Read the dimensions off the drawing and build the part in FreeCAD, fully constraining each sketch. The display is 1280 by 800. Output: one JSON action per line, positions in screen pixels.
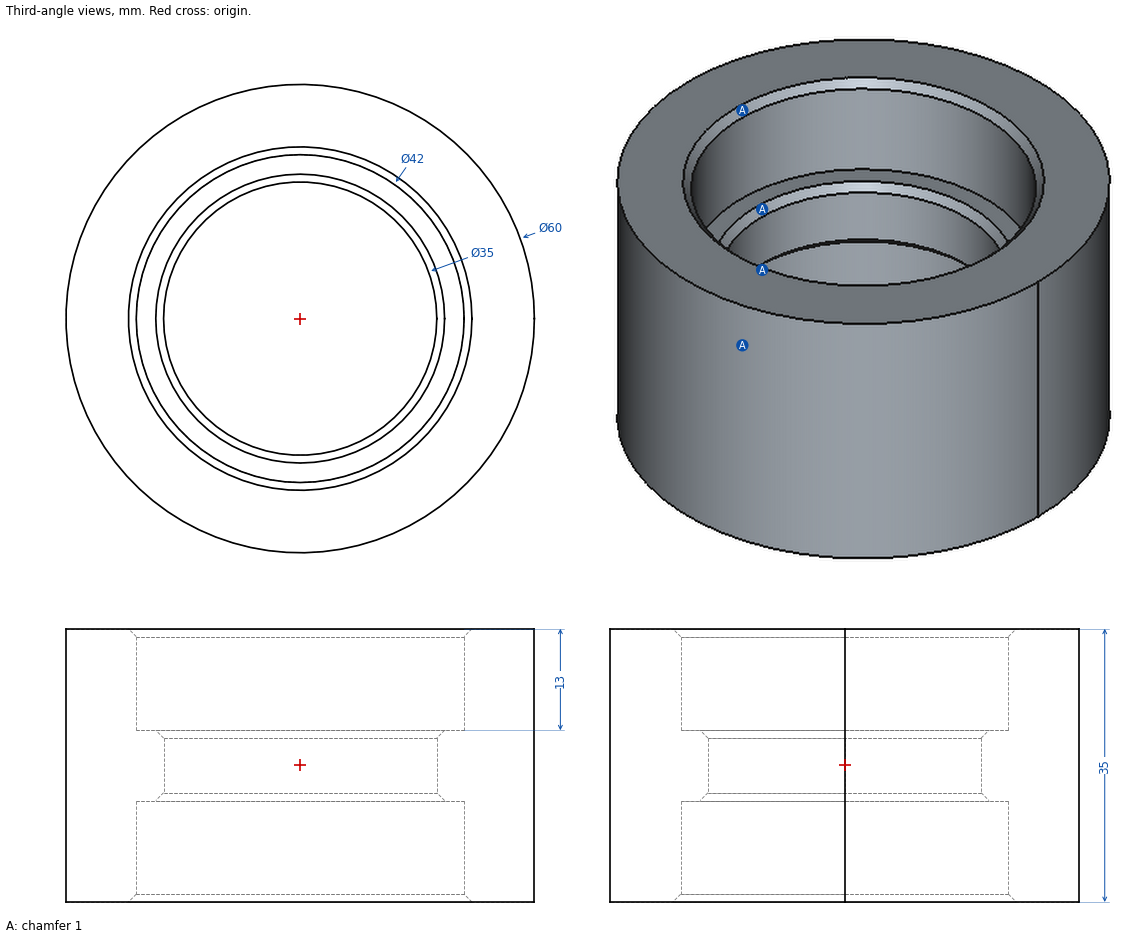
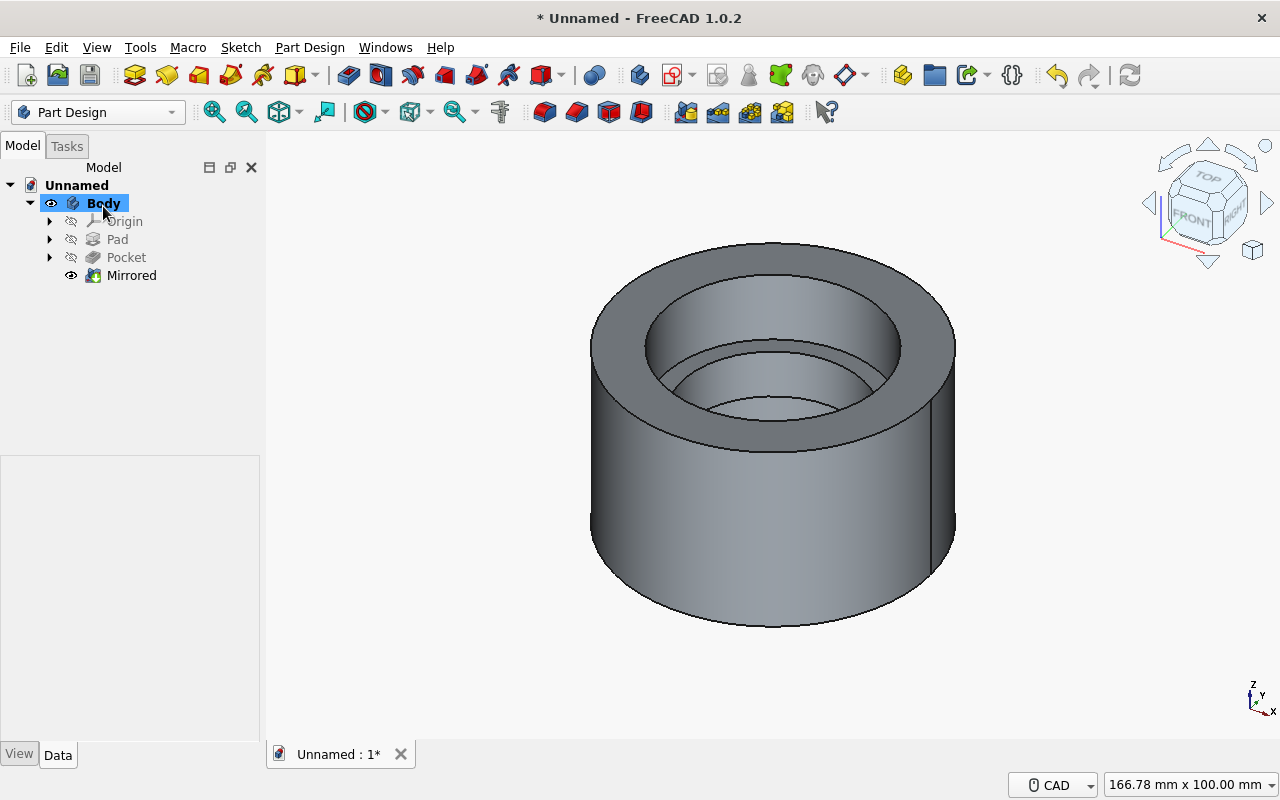
{"action": "left_click", "coordinate": [681, 381]}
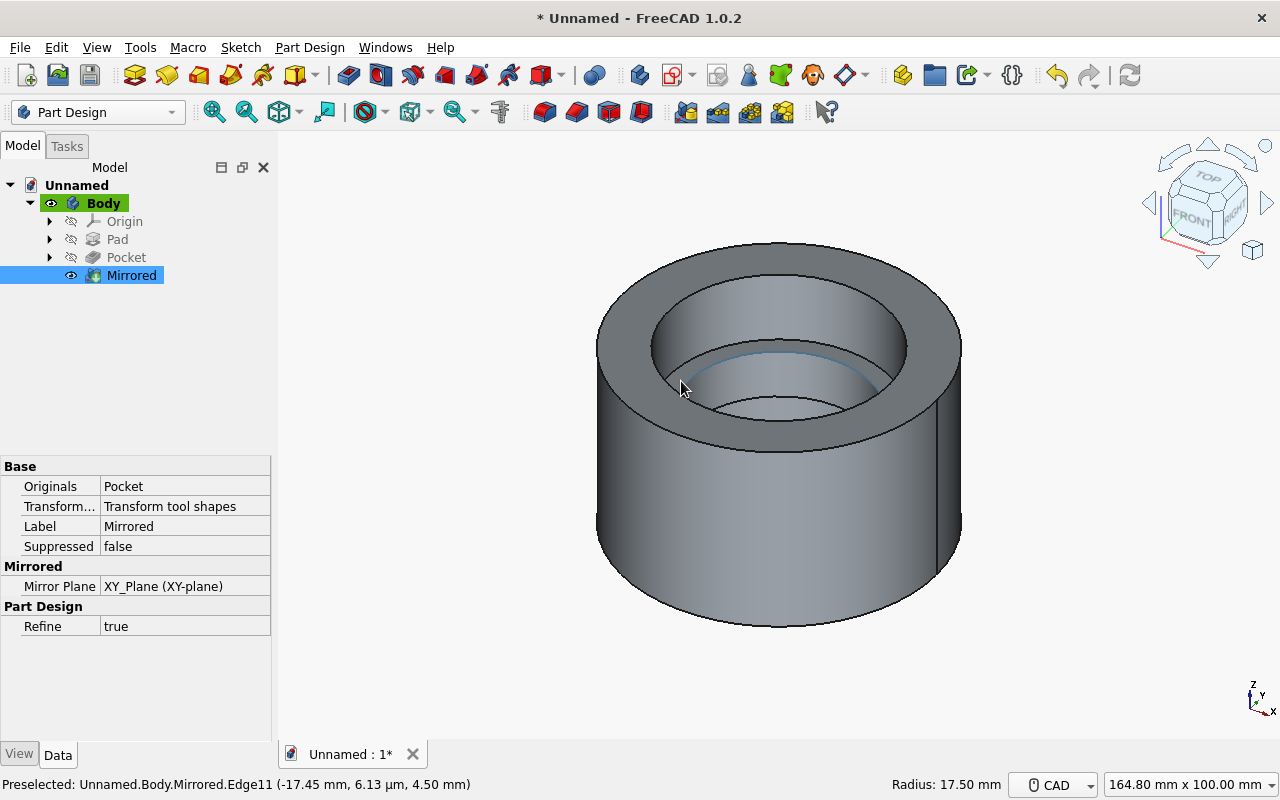
{"action": "left_click", "coordinate": [668, 310], "text": "ctrl"}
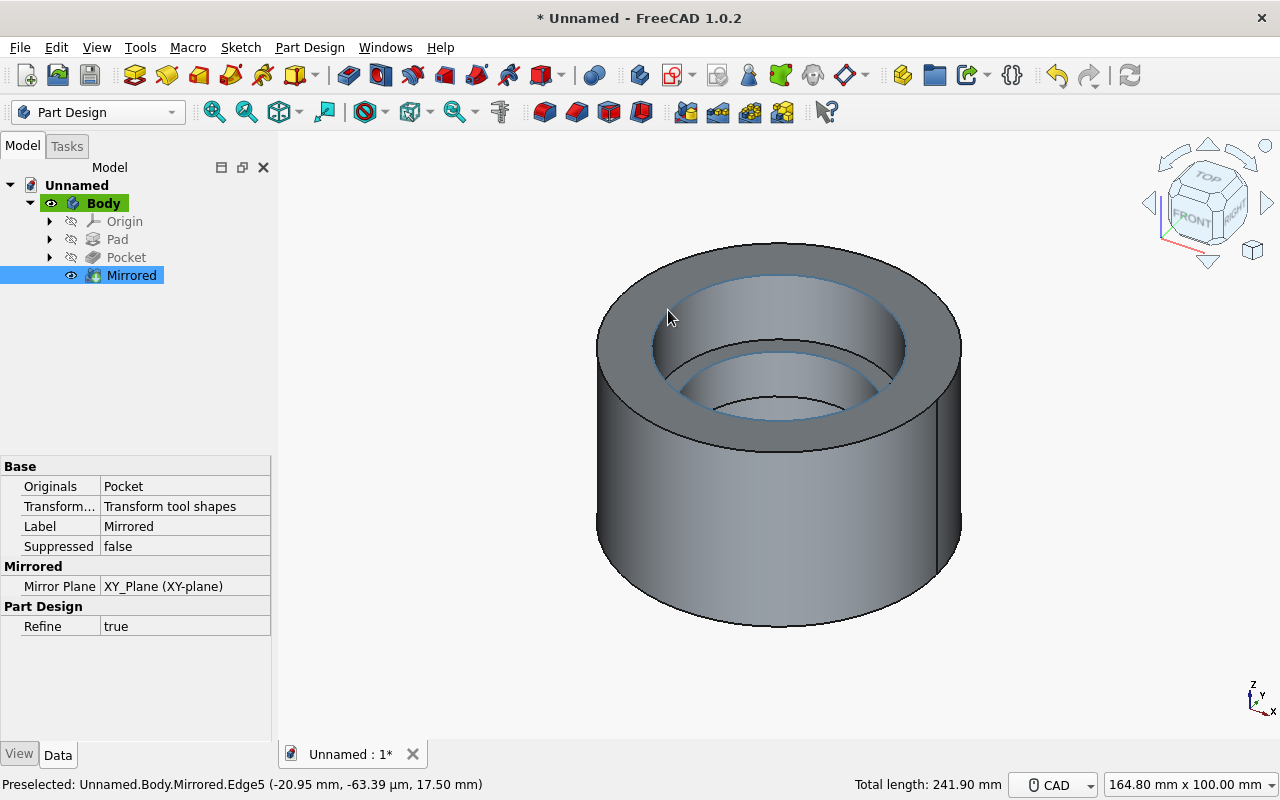
{"action": "key", "text": "0"}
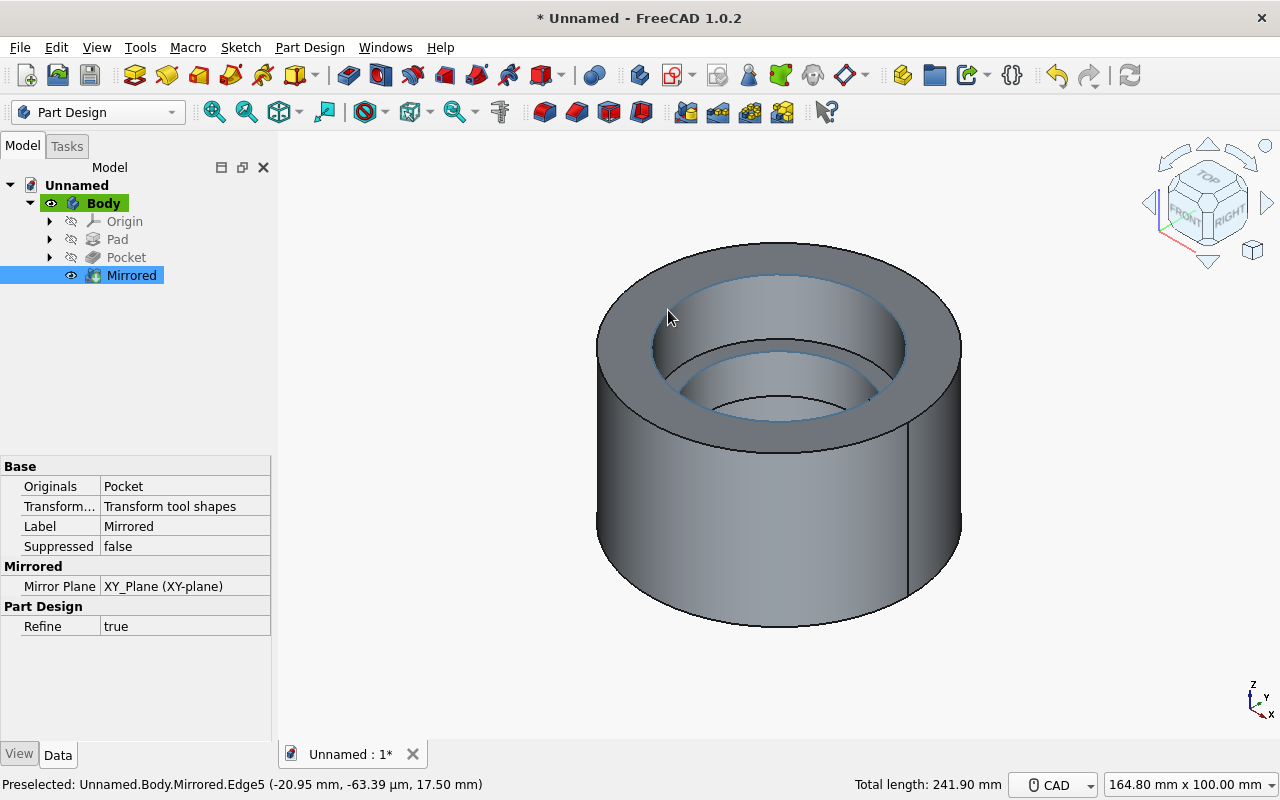
{"action": "key", "text": "2"}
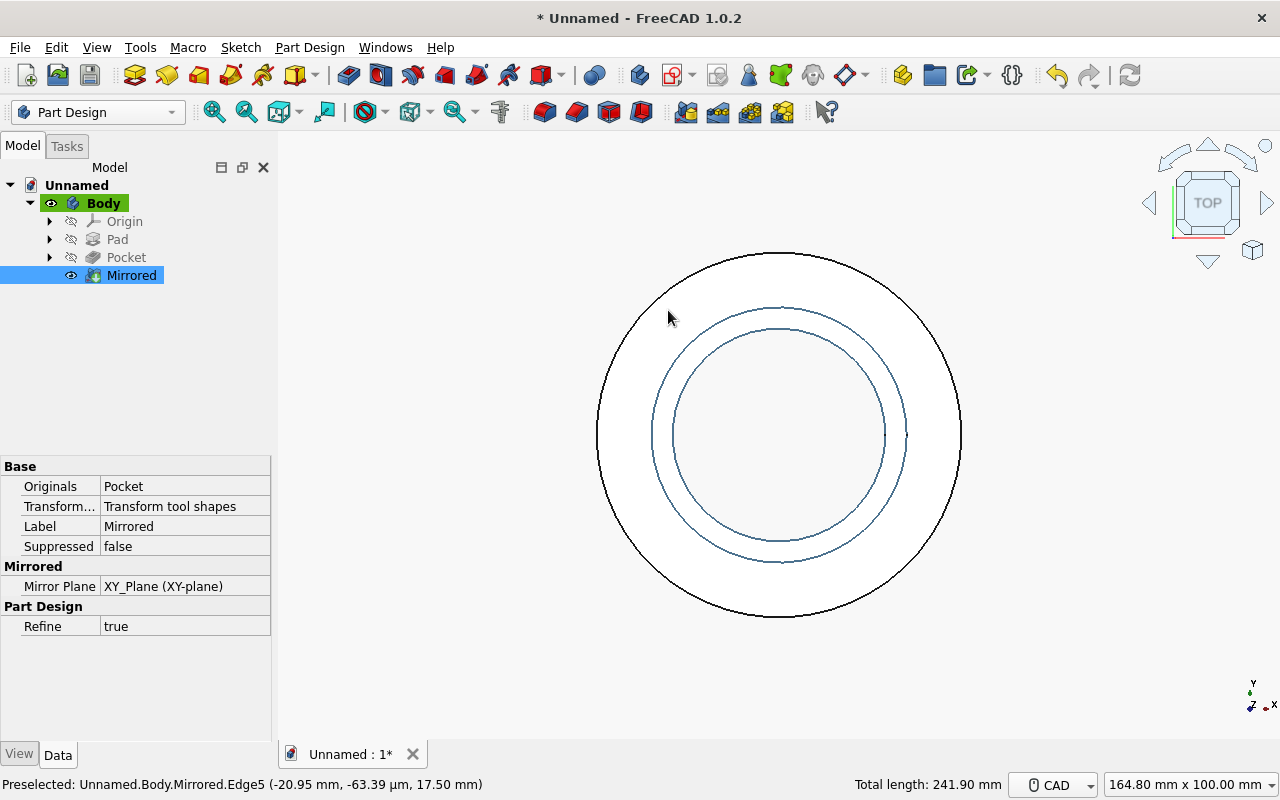
{"action": "key", "text": "1"}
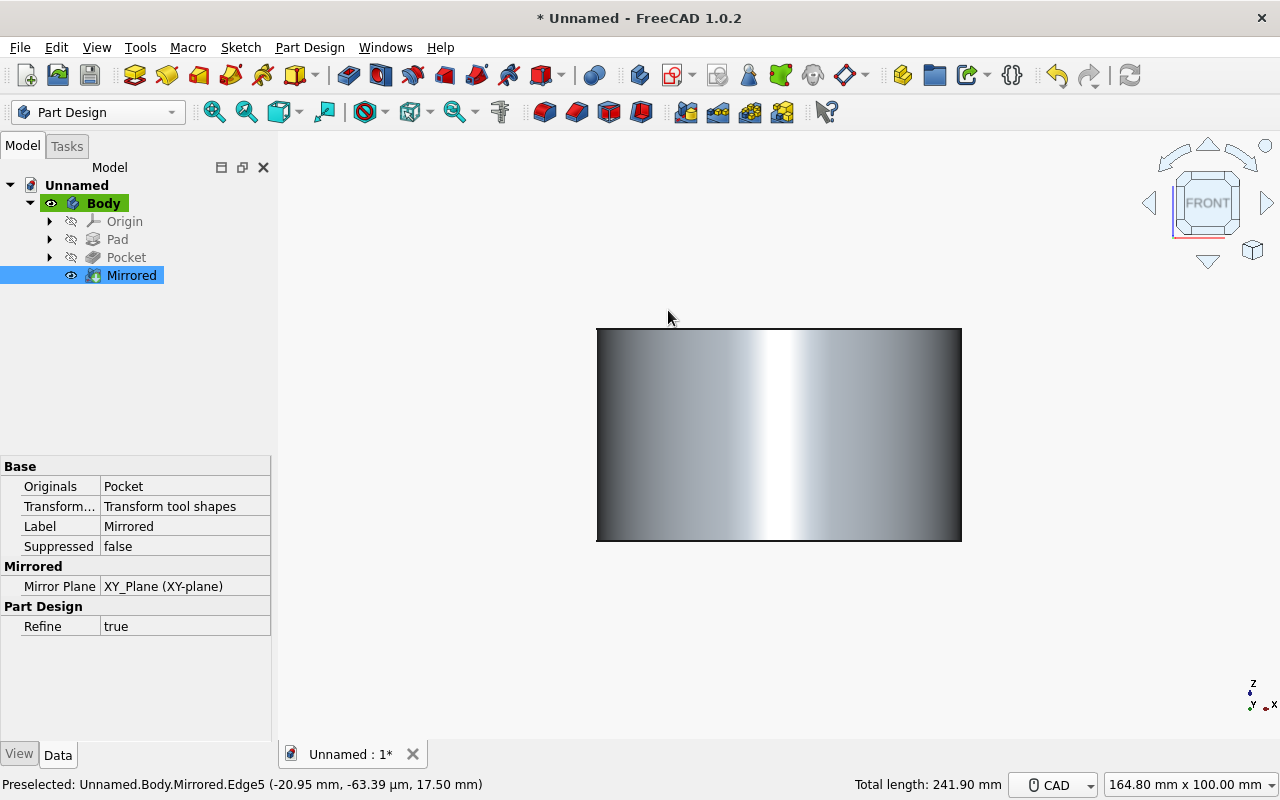
{"action": "left_click", "coordinate": [216, 112]}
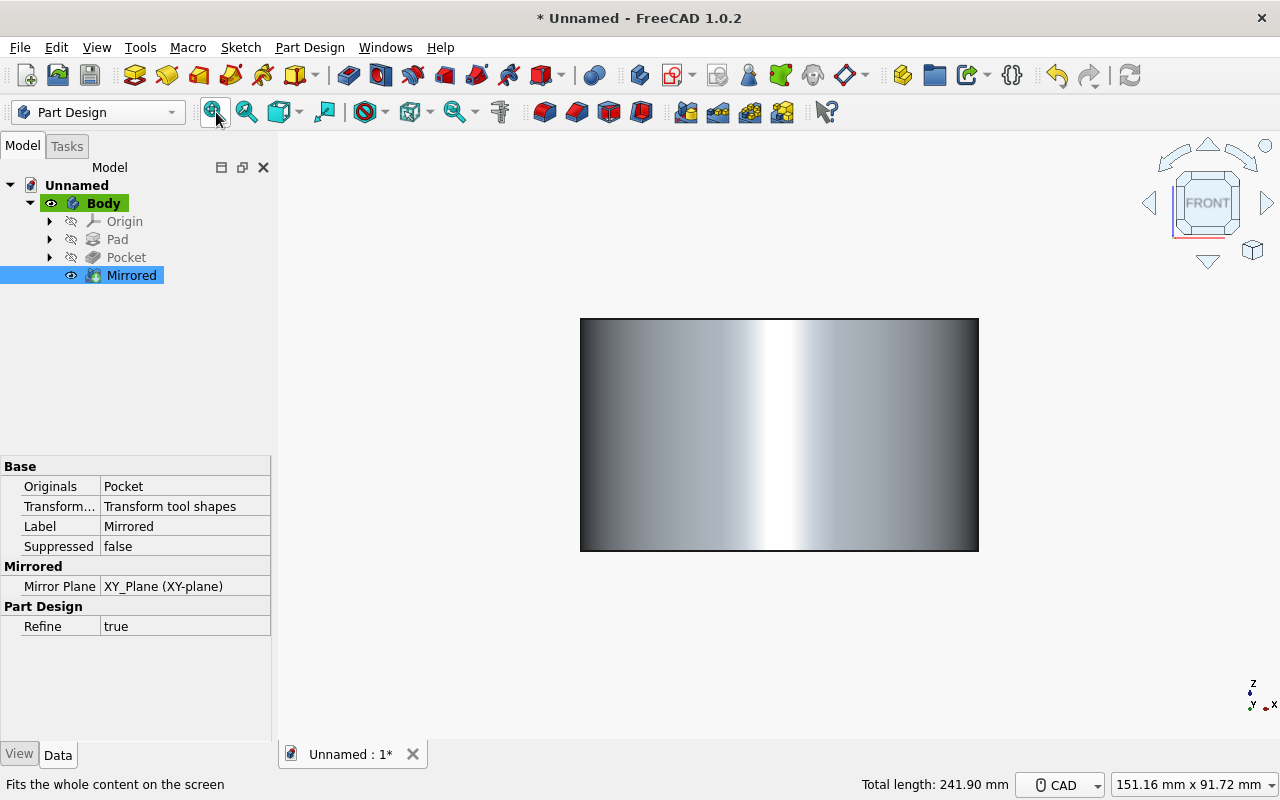
{"action": "key", "text": "3"}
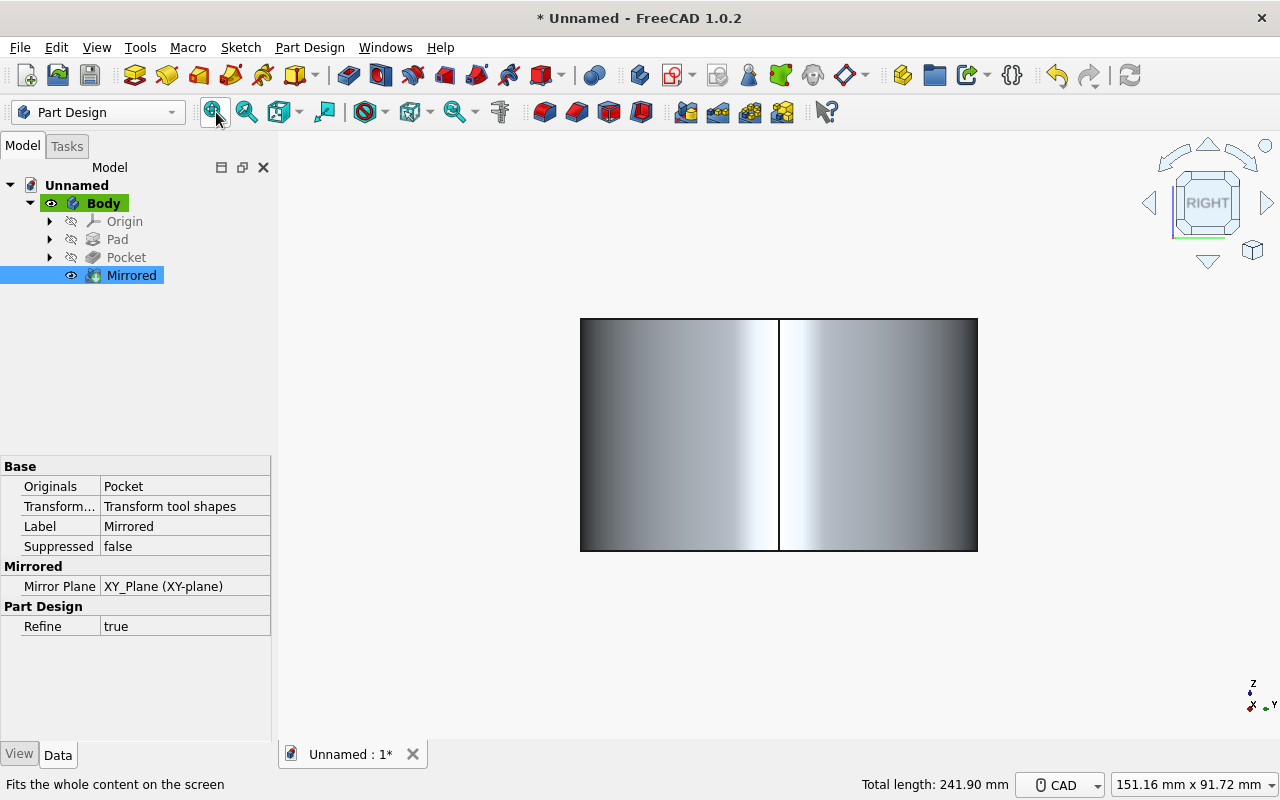
{"action": "left_click", "coordinate": [216, 112]}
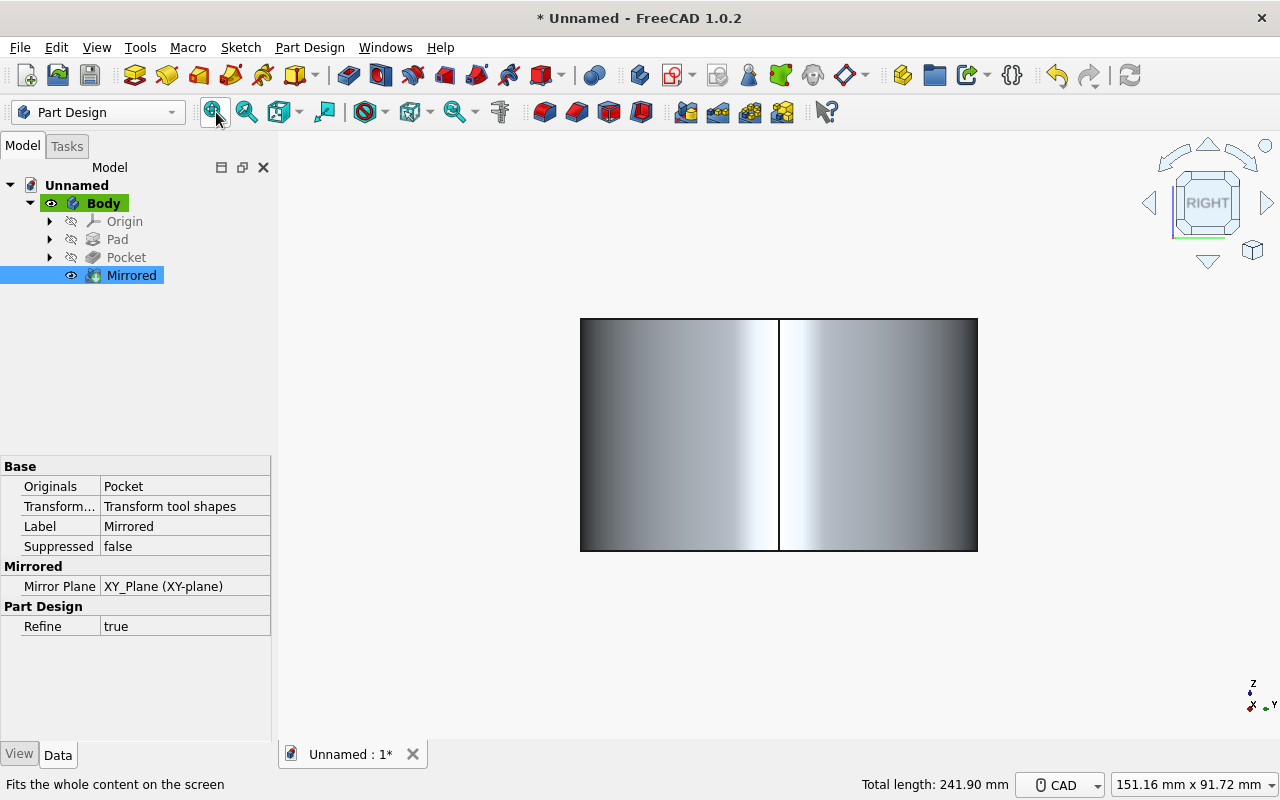
{"action": "key", "text": "5"}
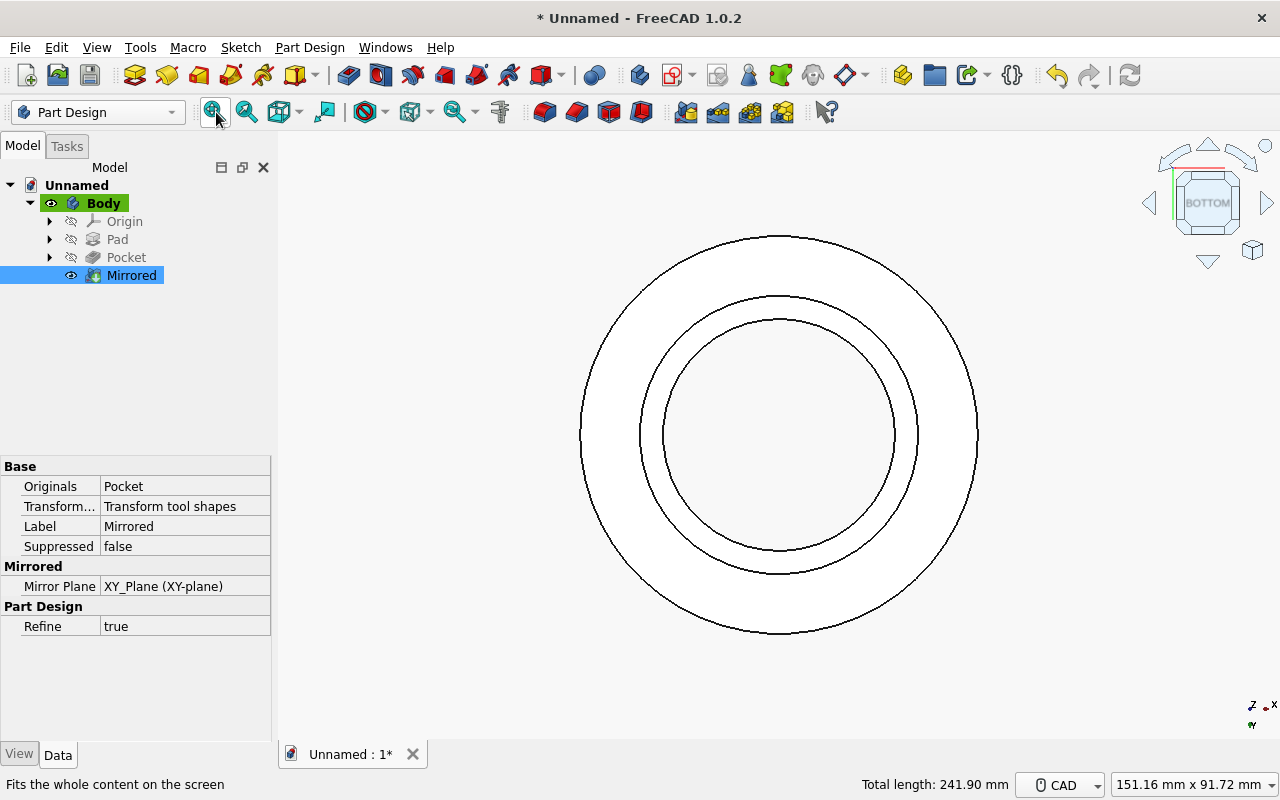
{"action": "left_click", "coordinate": [640, 434], "text": "ctrl"}